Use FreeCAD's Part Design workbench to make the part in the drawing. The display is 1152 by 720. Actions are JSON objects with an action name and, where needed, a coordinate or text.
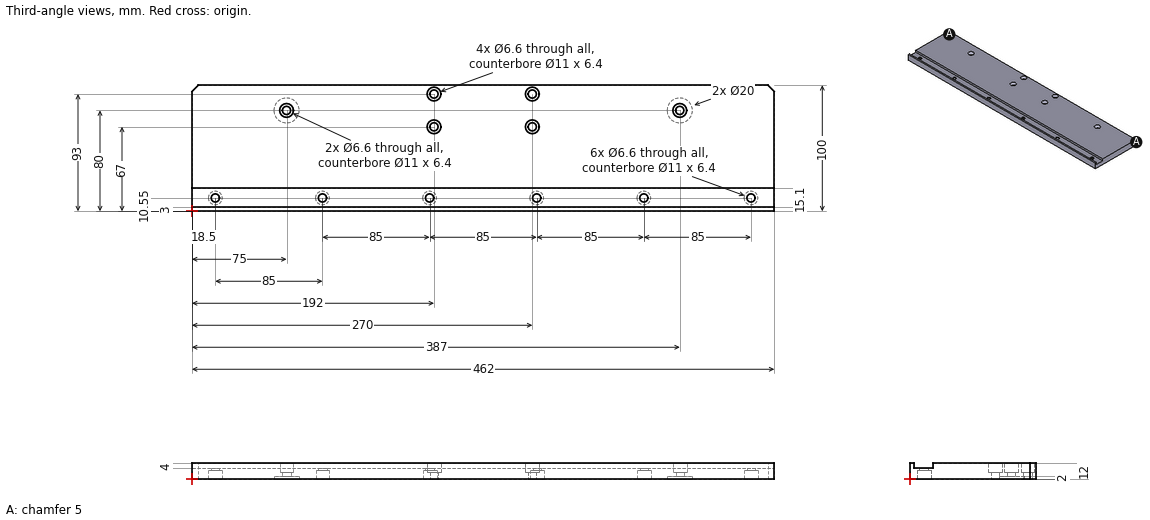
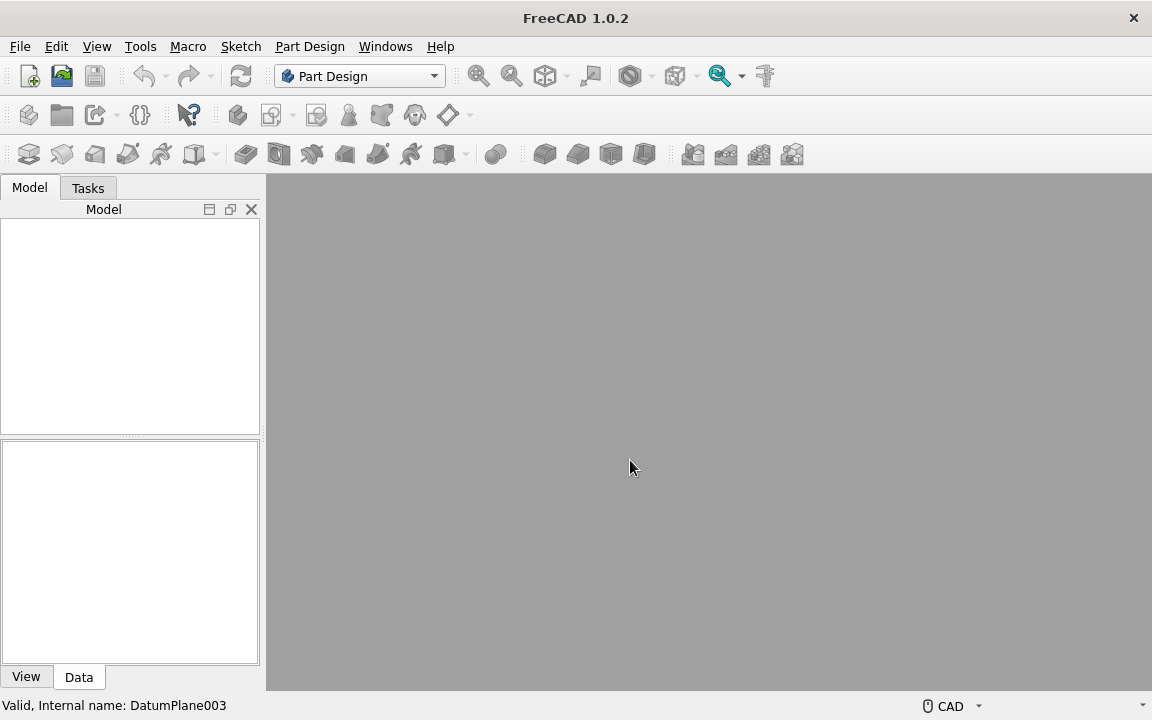
{"action": "left_click", "coordinate": [29, 76]}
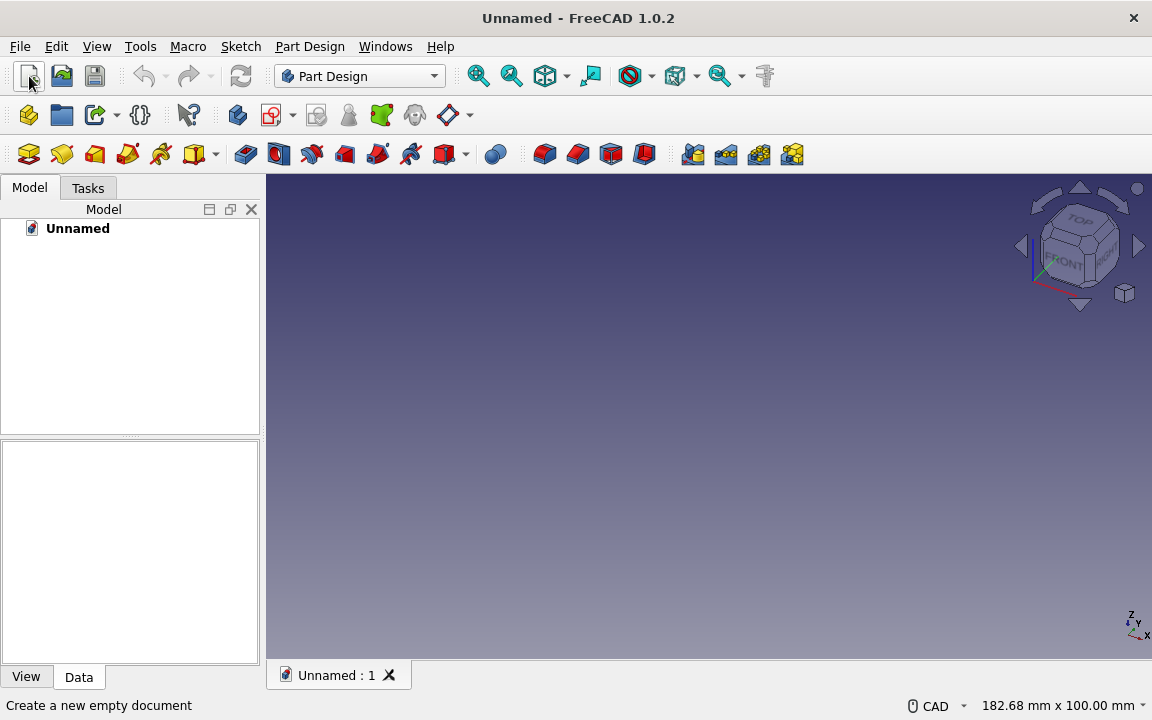
{"action": "left_click", "coordinate": [270, 116]}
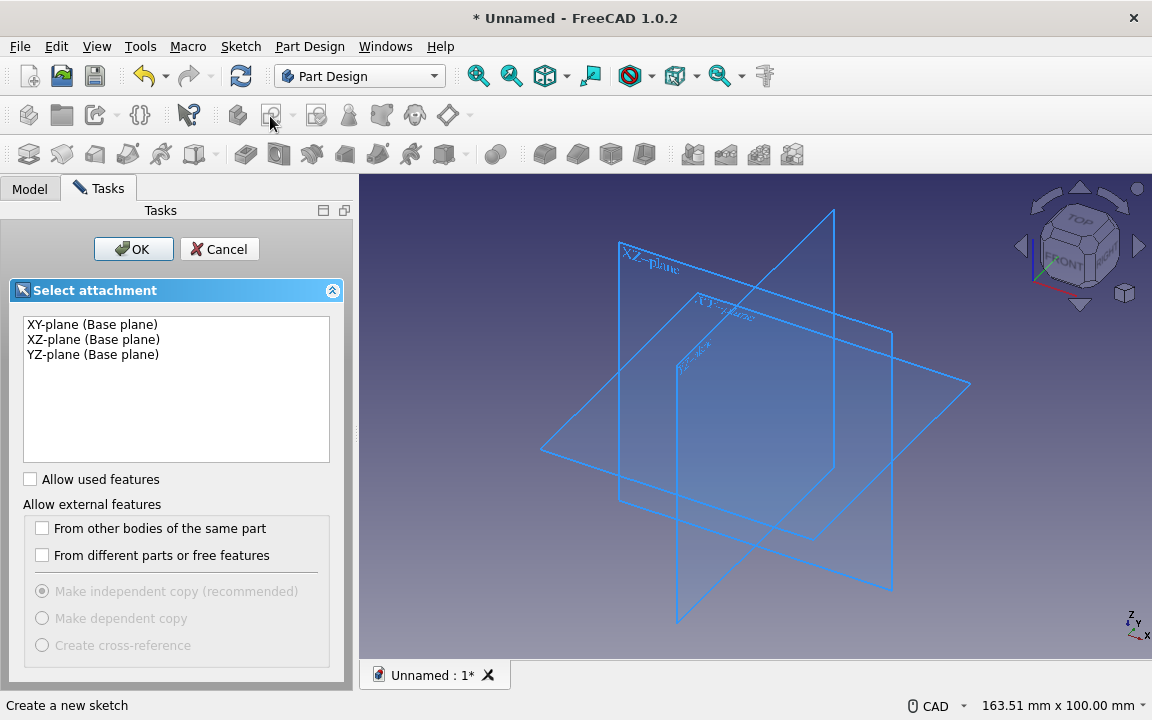
{"action": "left_click", "coordinate": [84, 324]}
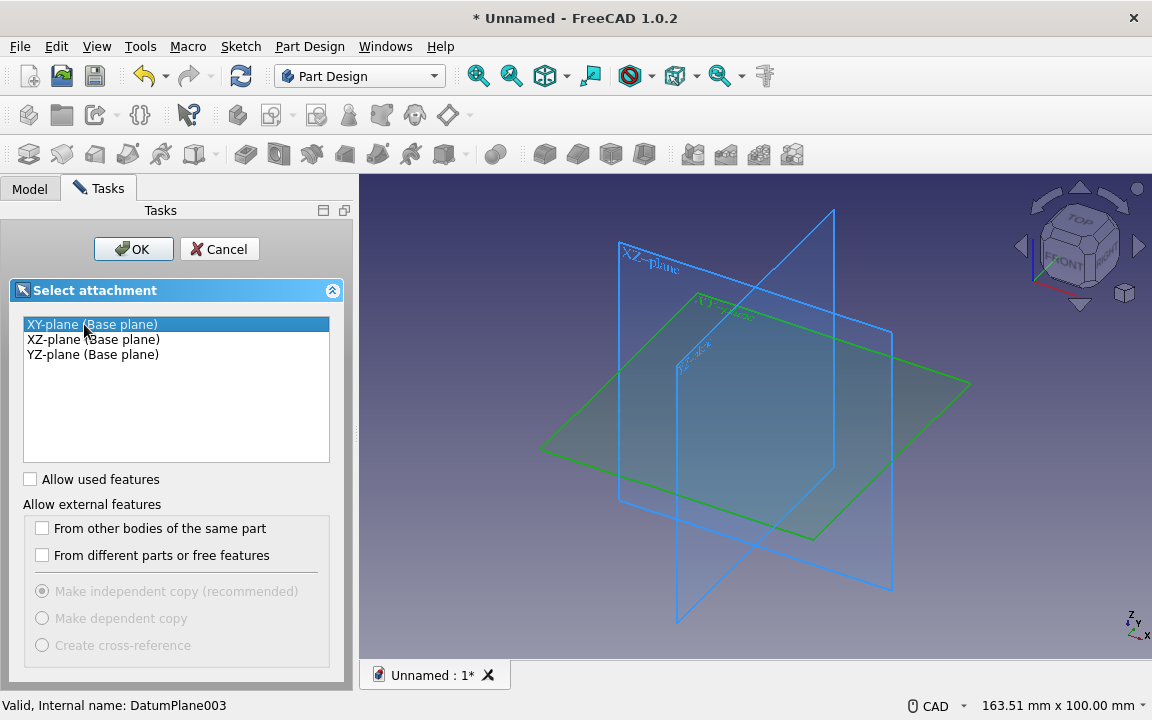
{"action": "left_click", "coordinate": [134, 249]}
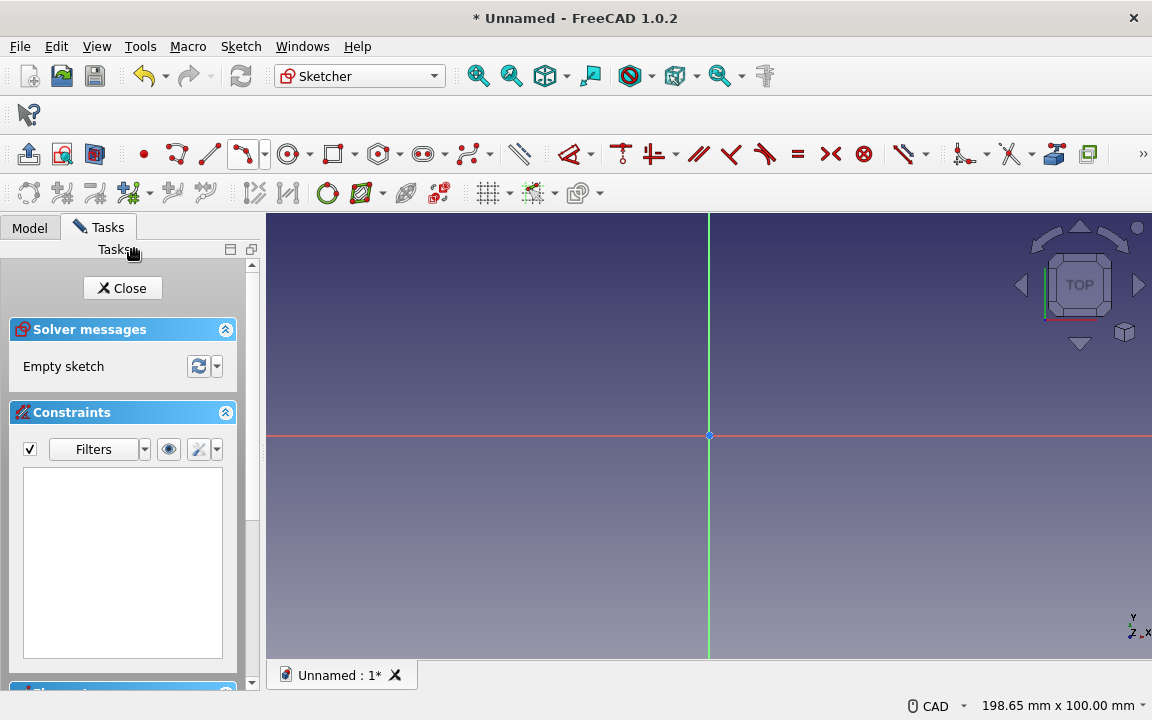
{"action": "scroll", "coordinate": [294, 509], "scroll_direction": "down", "scroll_amount": 7}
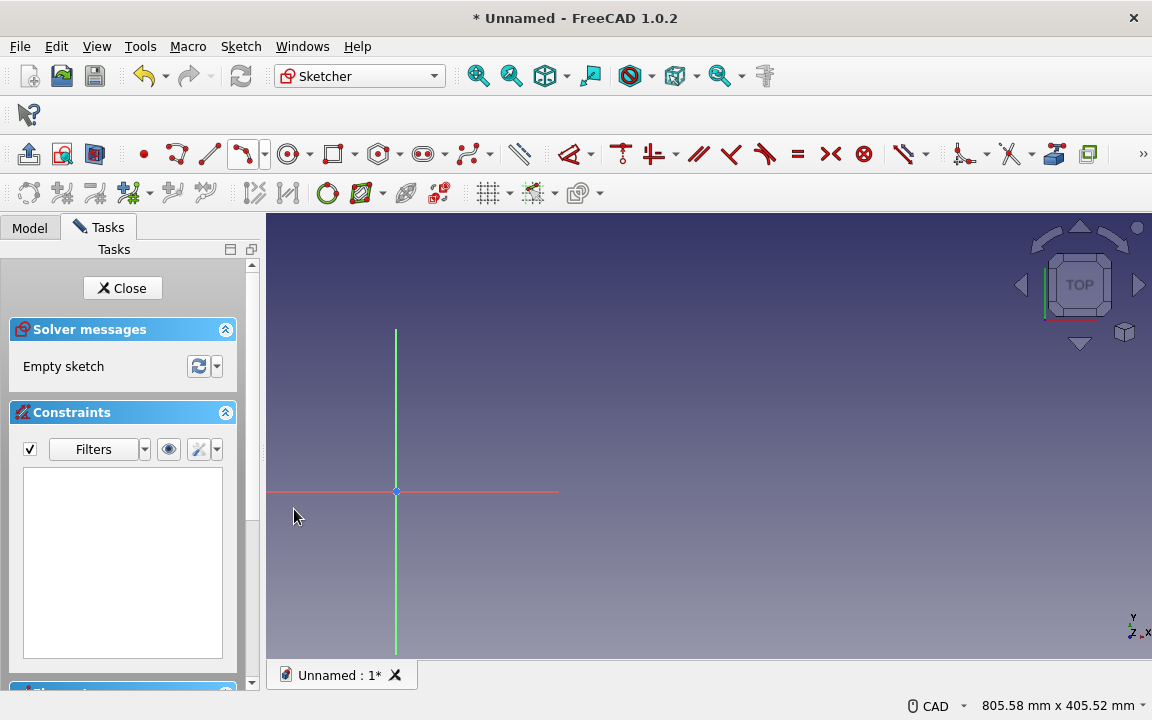
{"action": "left_click", "coordinate": [332, 154]}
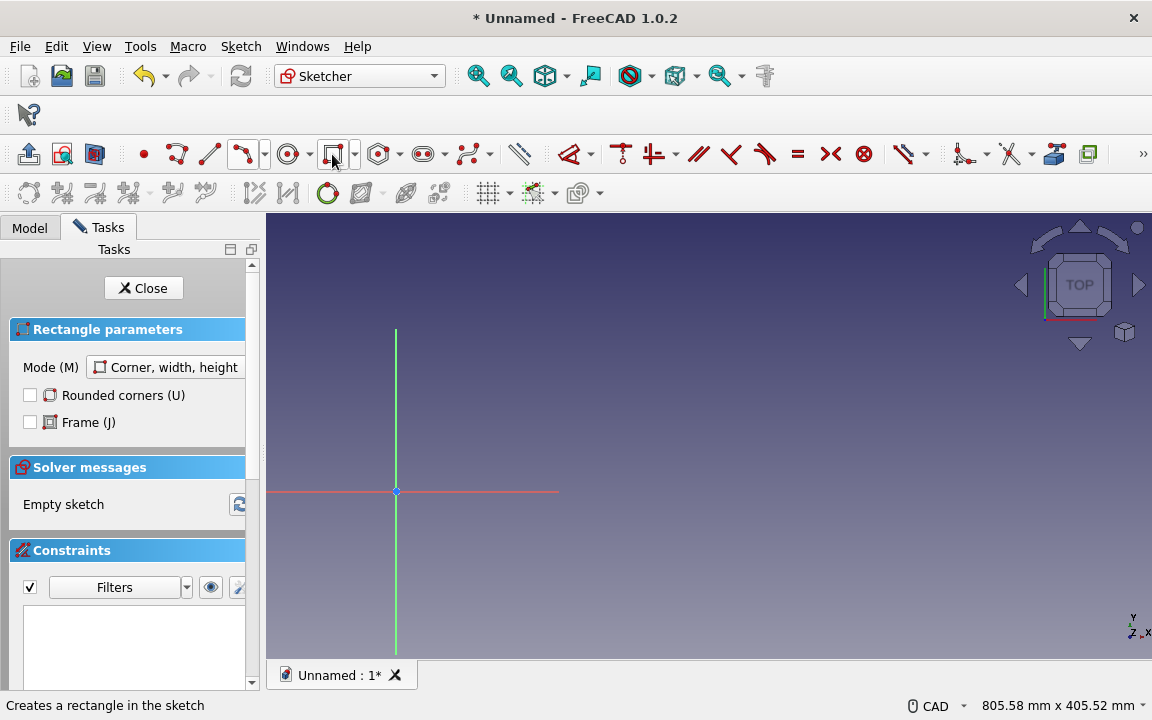
{"action": "left_click", "coordinate": [396, 491]}
{"action": "mouse_move", "coordinate": [904, 382]}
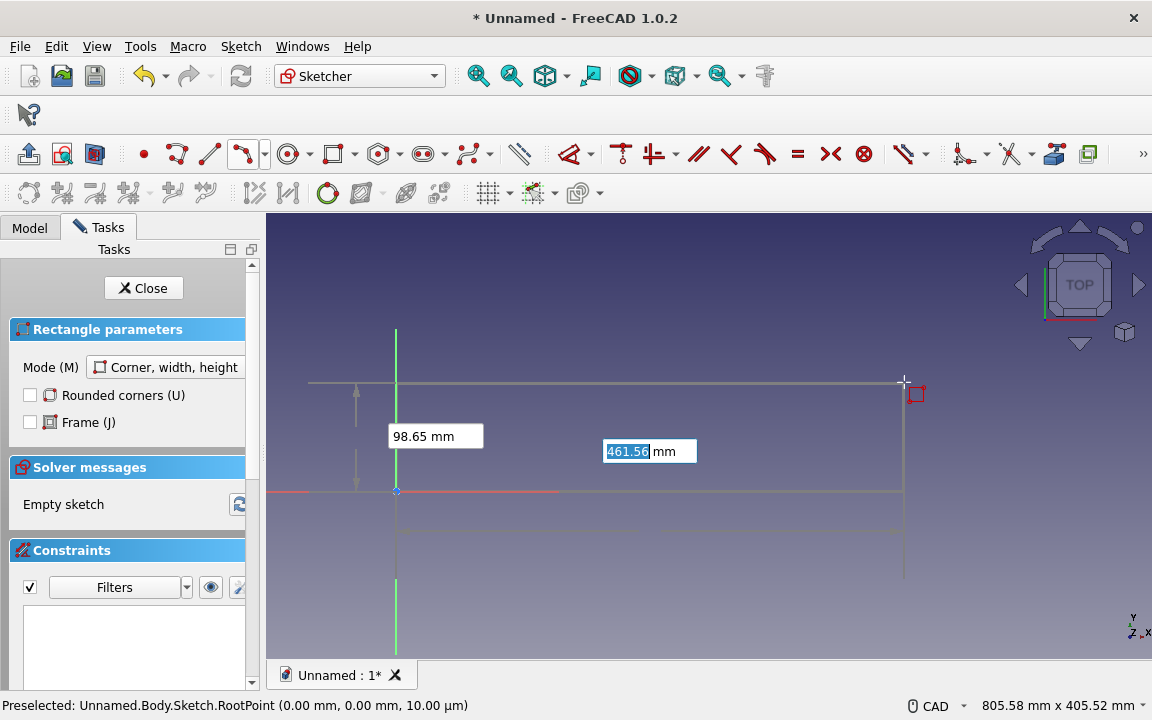
{"action": "type", "text": "462"}
{"action": "key", "text": "Tab"}
{"action": "type", "text": "100"}
{"action": "key", "text": "Return"}
{"action": "key", "text": "Escape"}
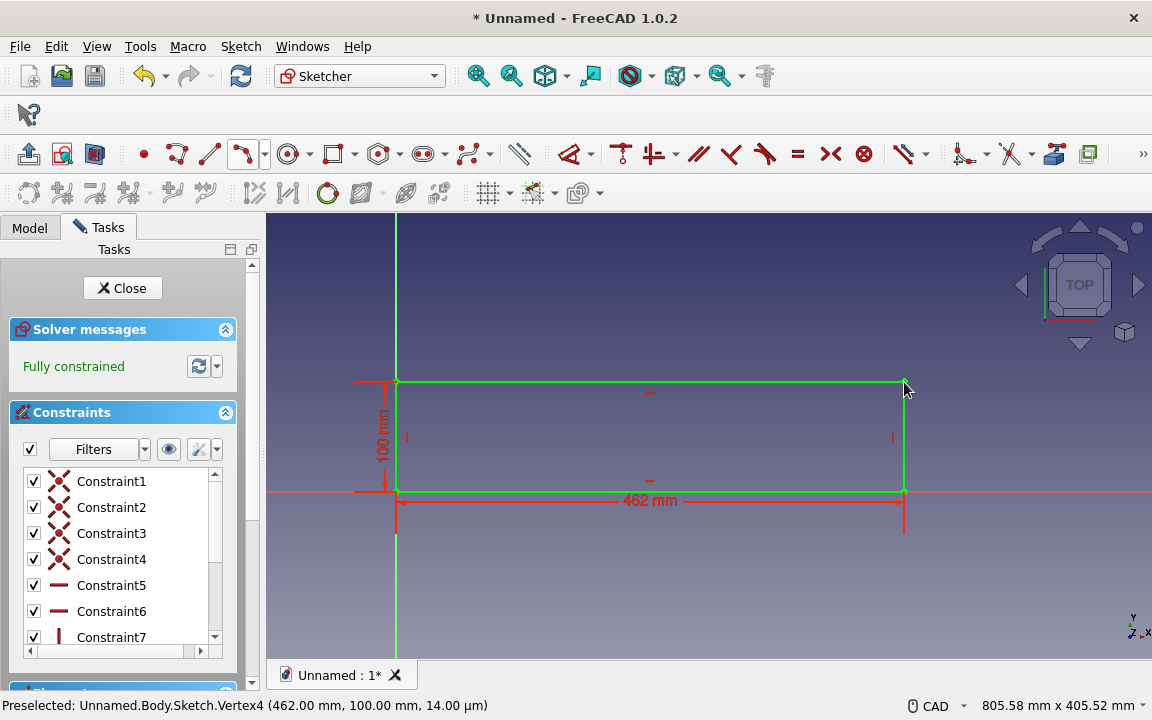
{"action": "left_click", "coordinate": [123, 288]}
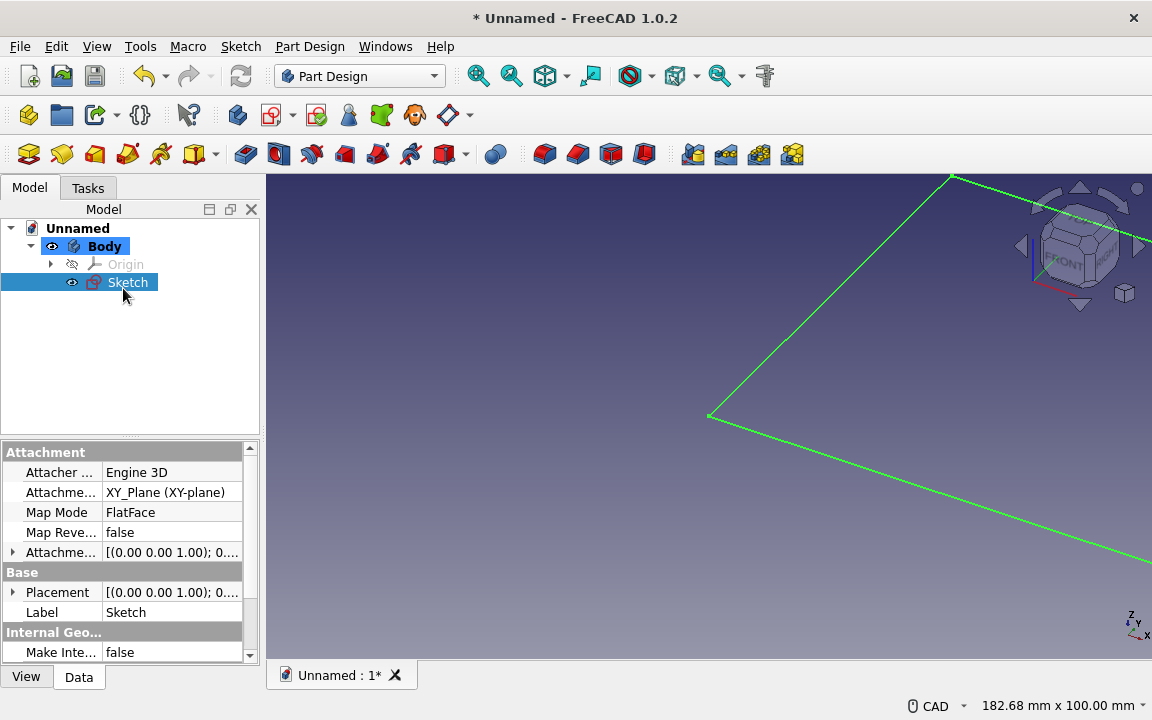
{"action": "left_click", "coordinate": [29, 154]}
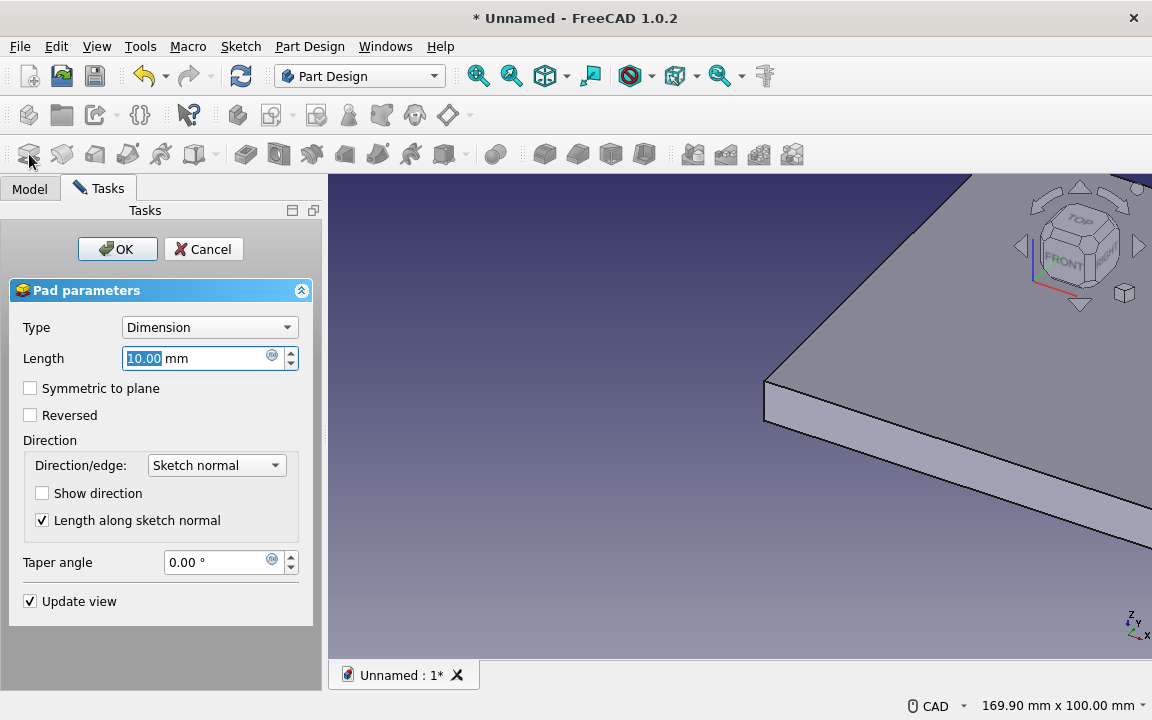
{"action": "type", "text": "12"}
{"action": "key", "text": "Tab"}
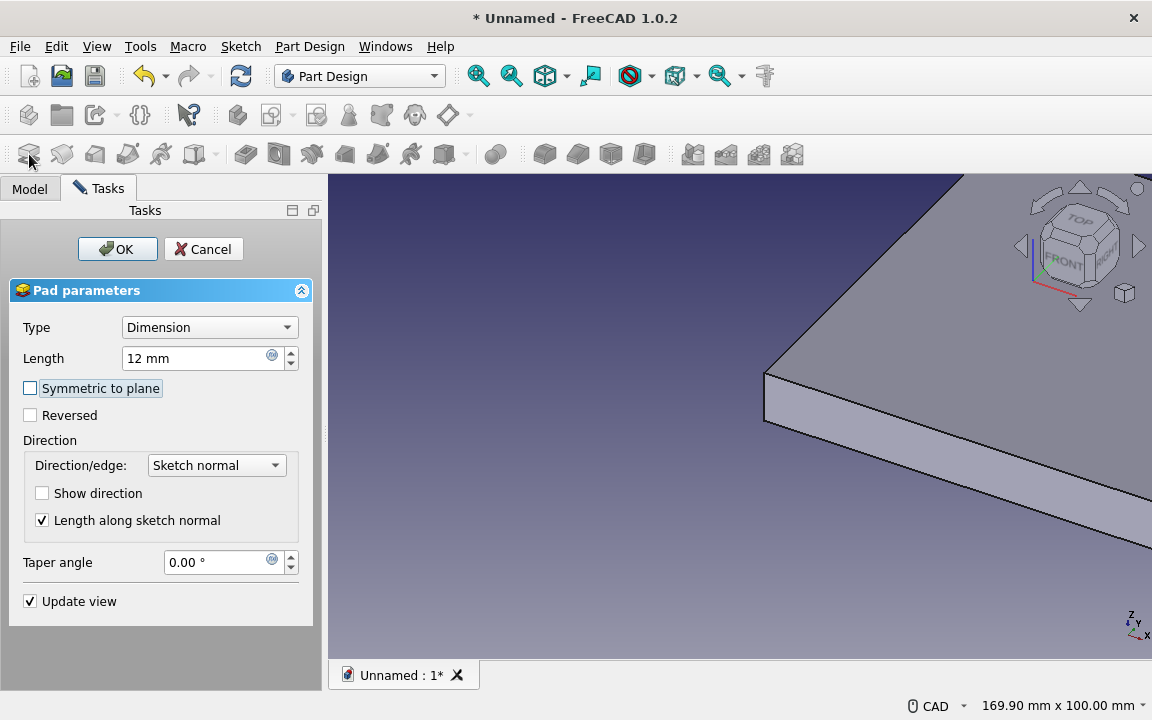
{"action": "left_click", "coordinate": [118, 249]}